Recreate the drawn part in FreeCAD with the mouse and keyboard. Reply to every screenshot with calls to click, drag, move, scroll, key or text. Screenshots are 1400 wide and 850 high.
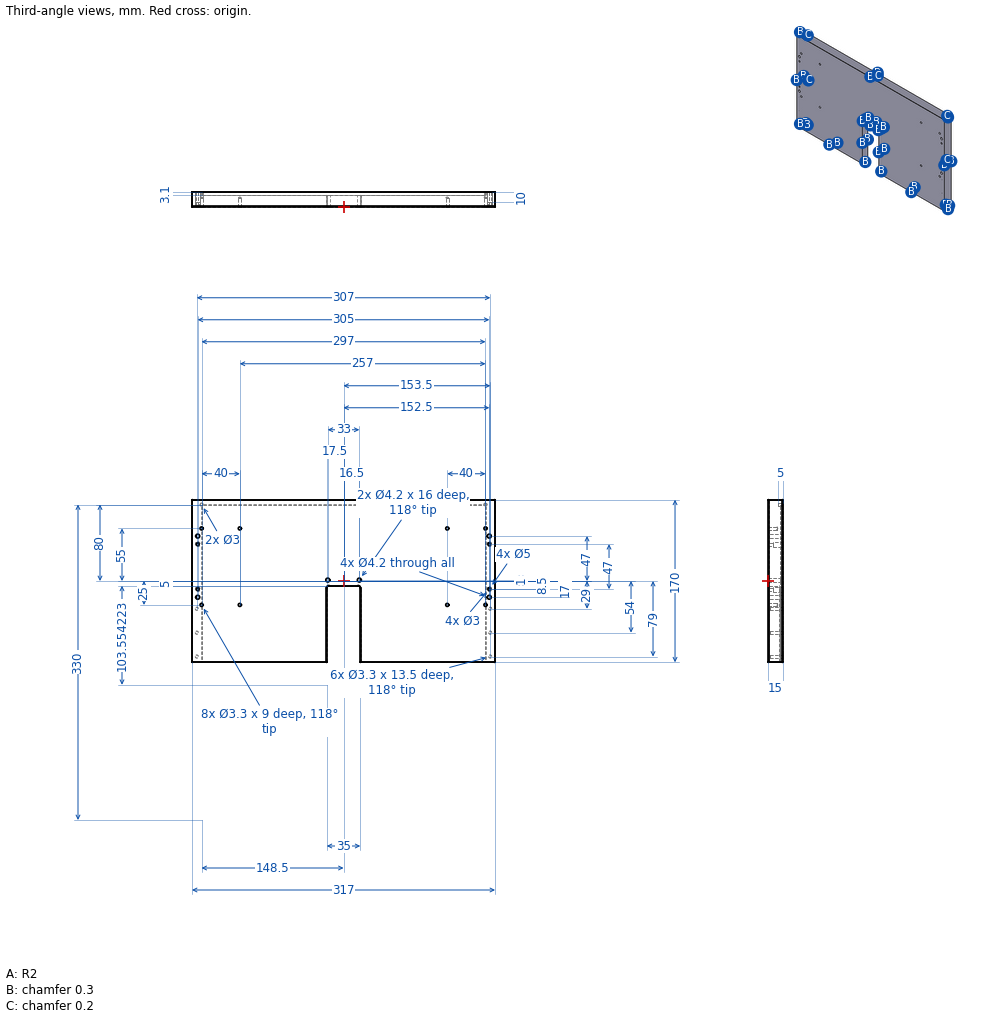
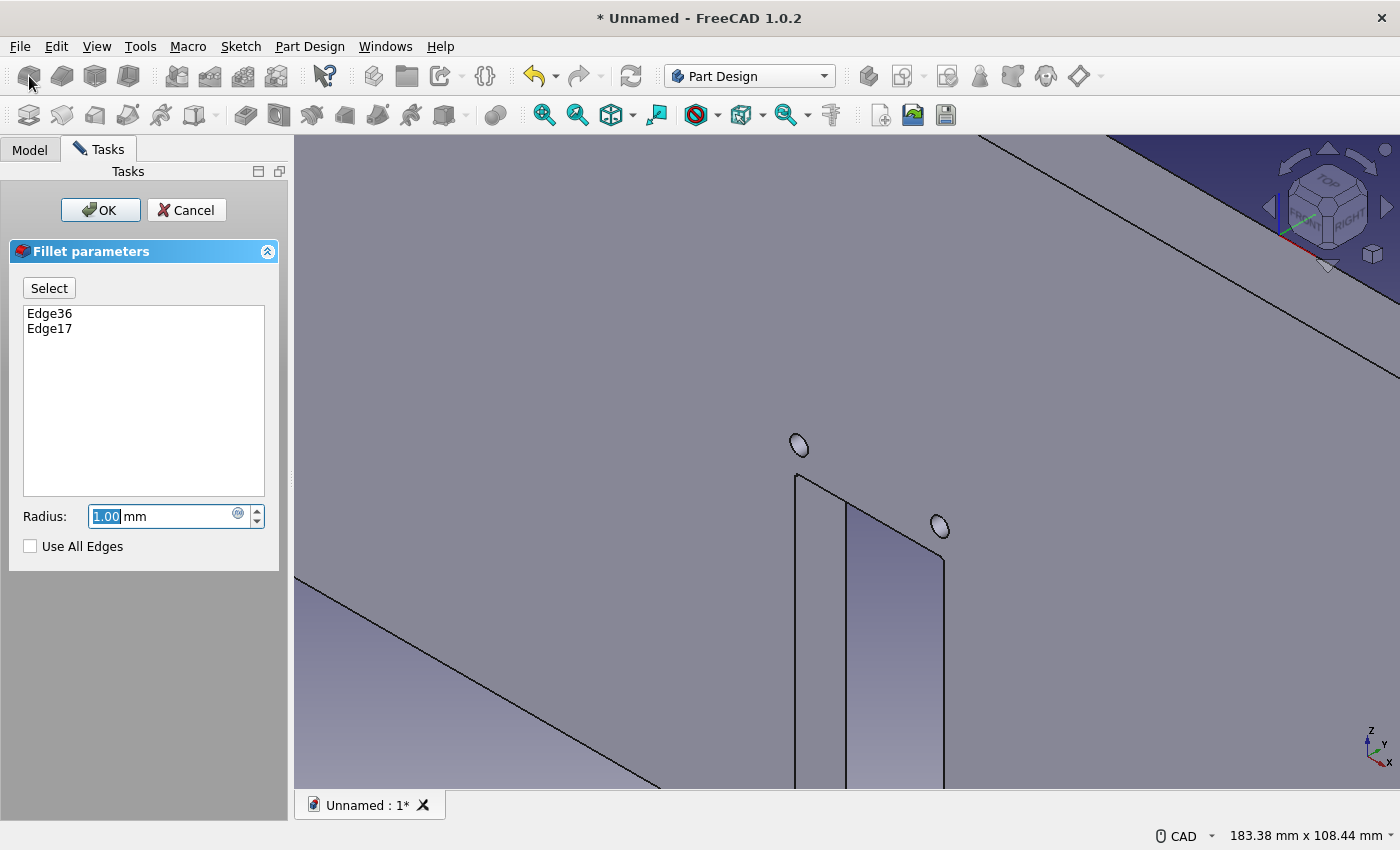
text(2)
key(Tab)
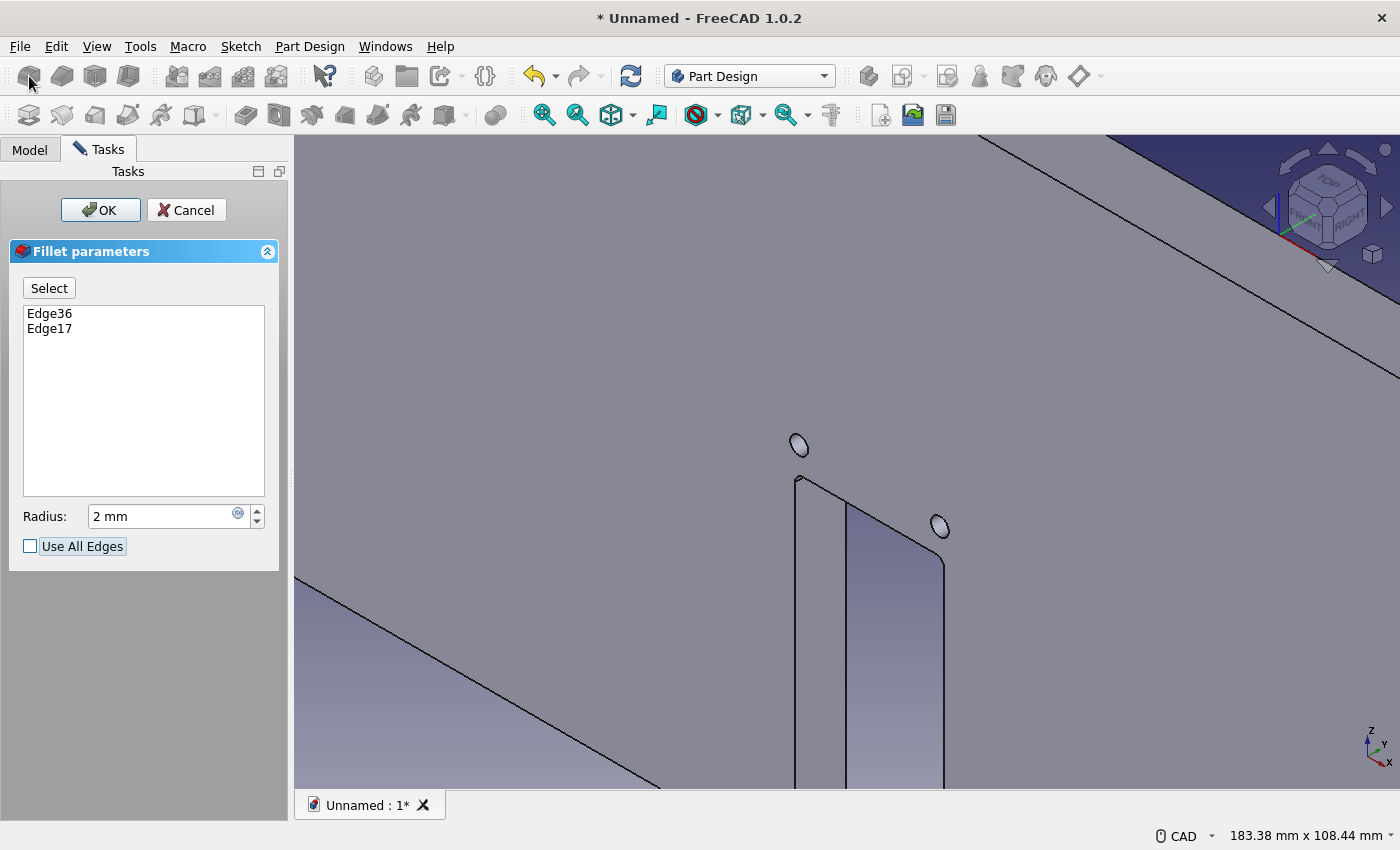
click(101, 210)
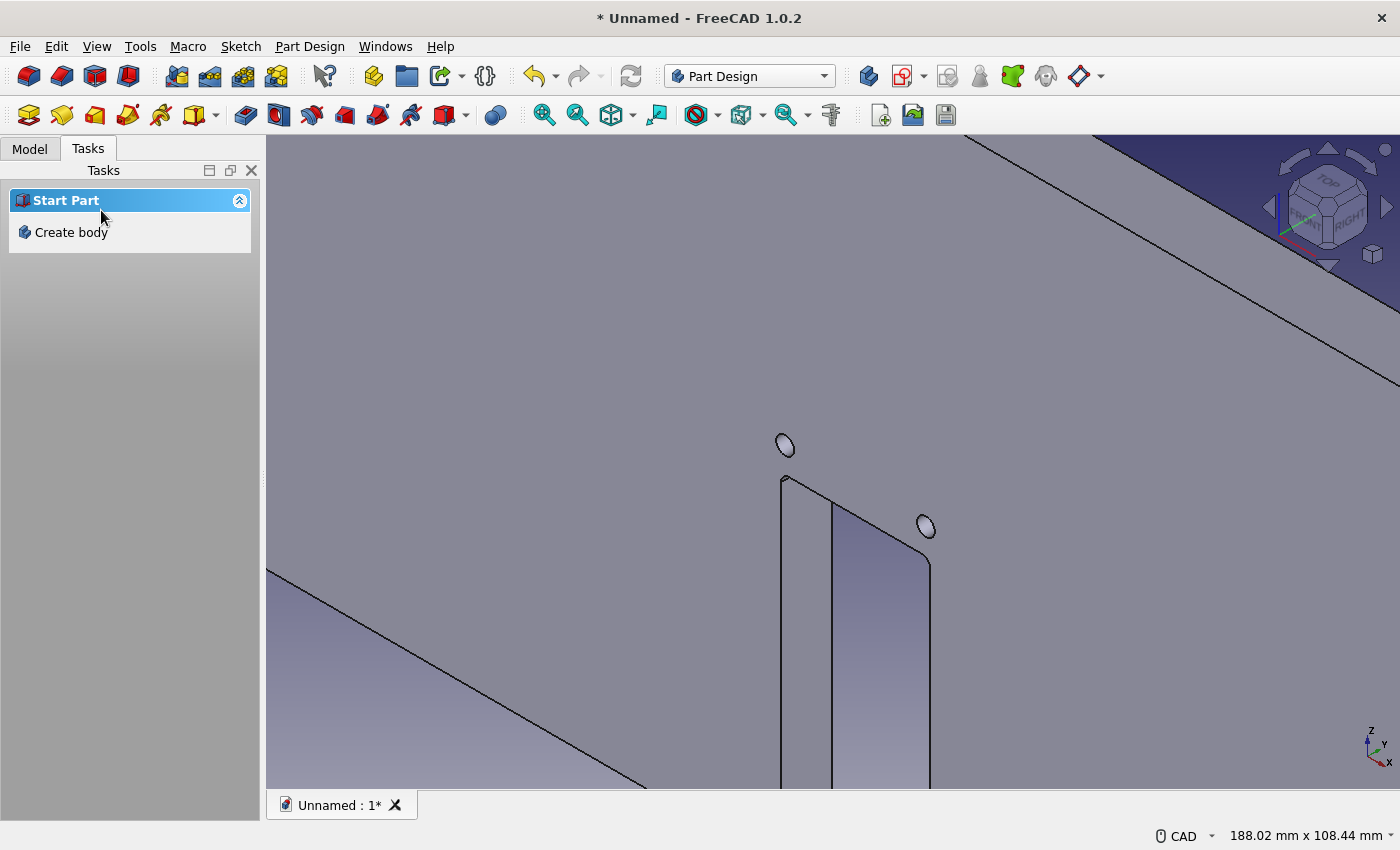
key(v)
key(f)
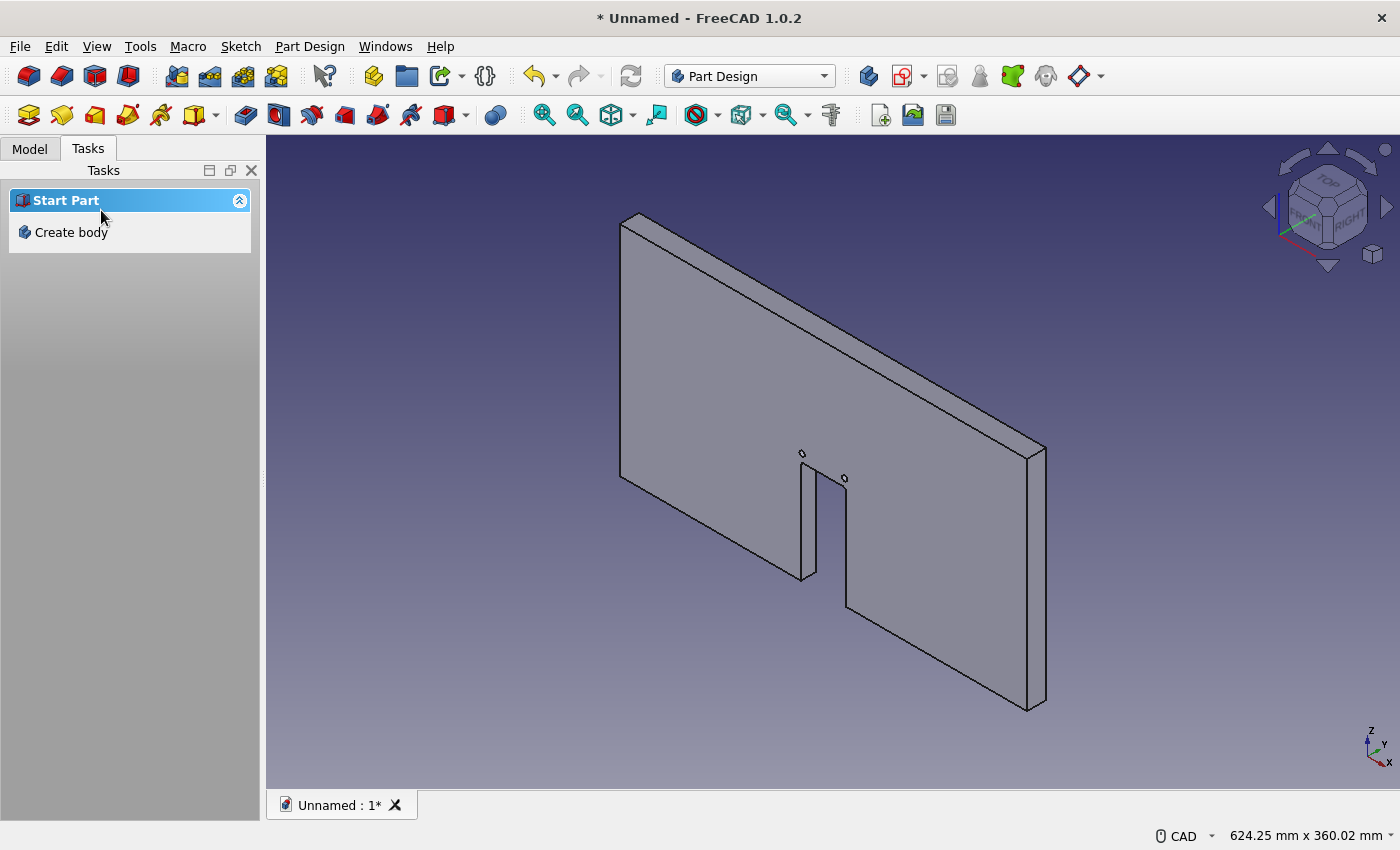
key(4)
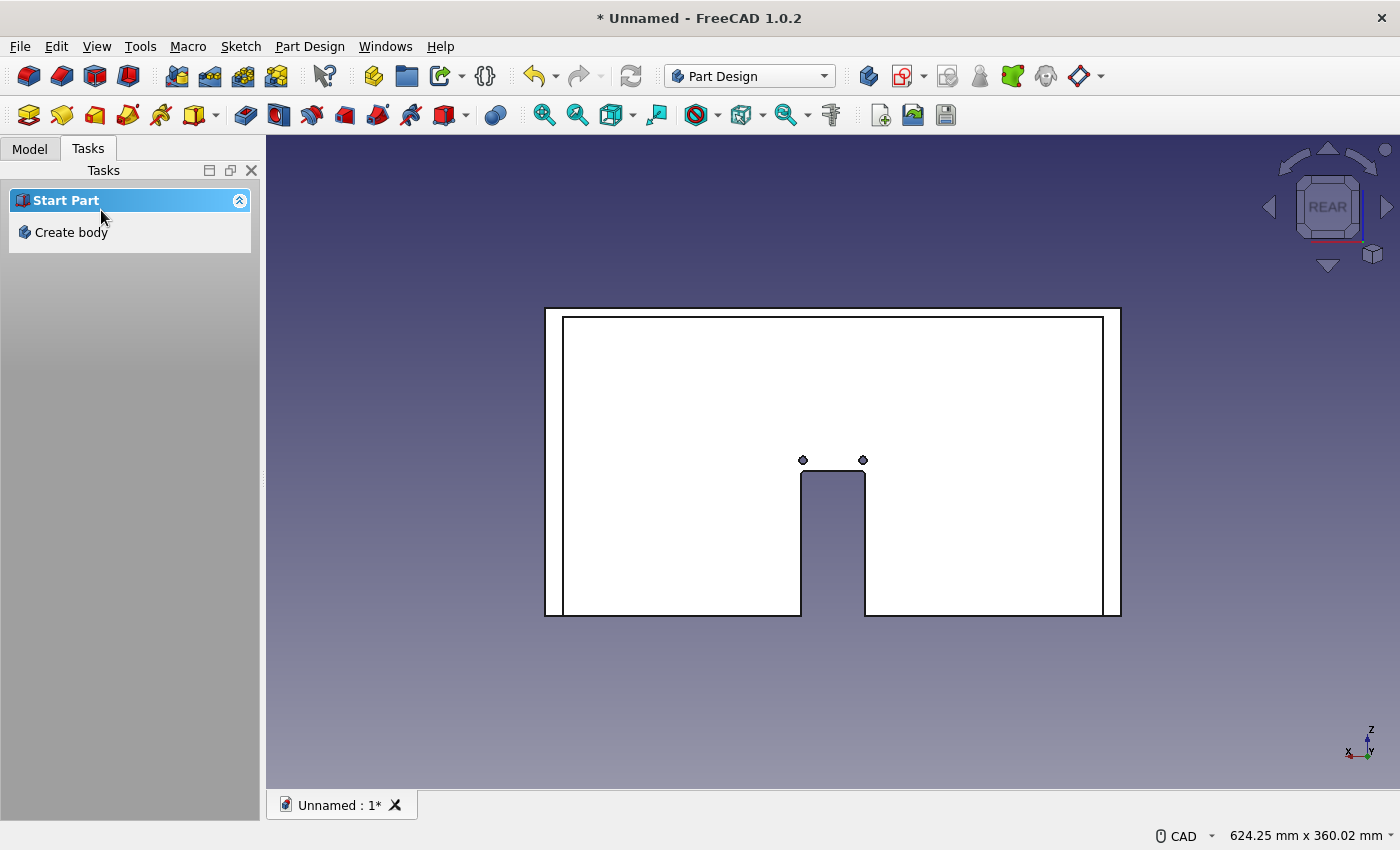
scroll(551, 413, up, 4)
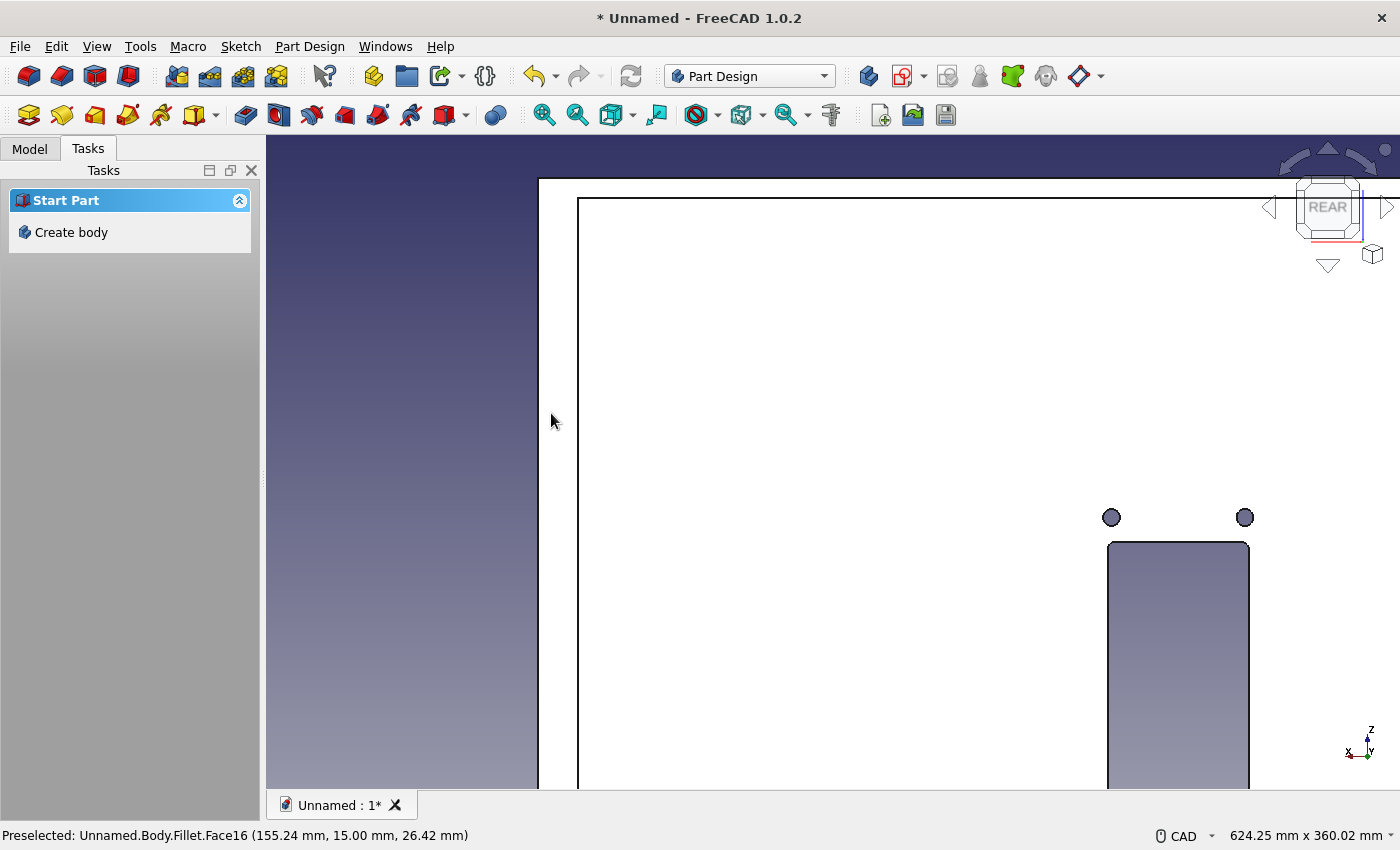
click(551, 413)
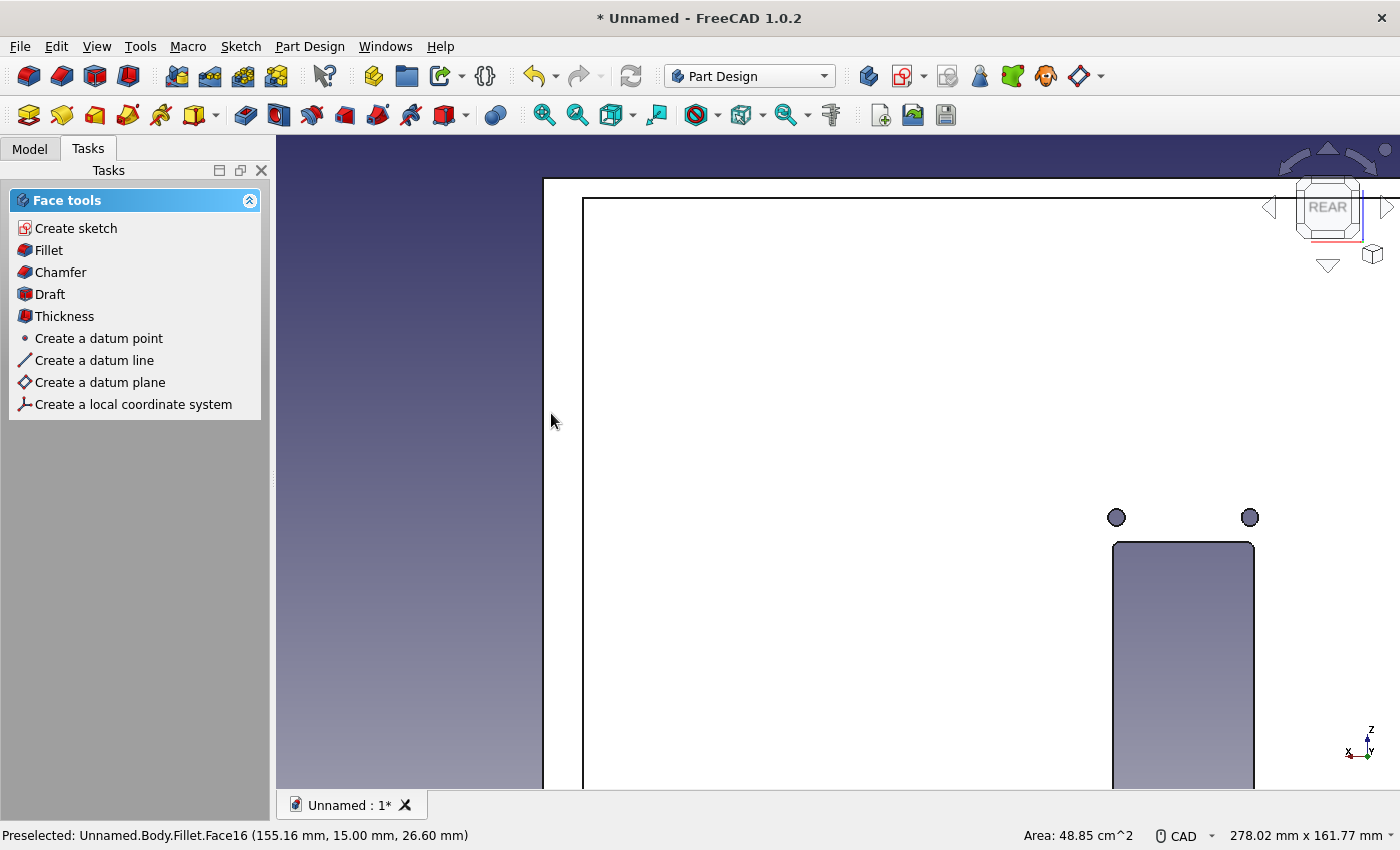
click(902, 76)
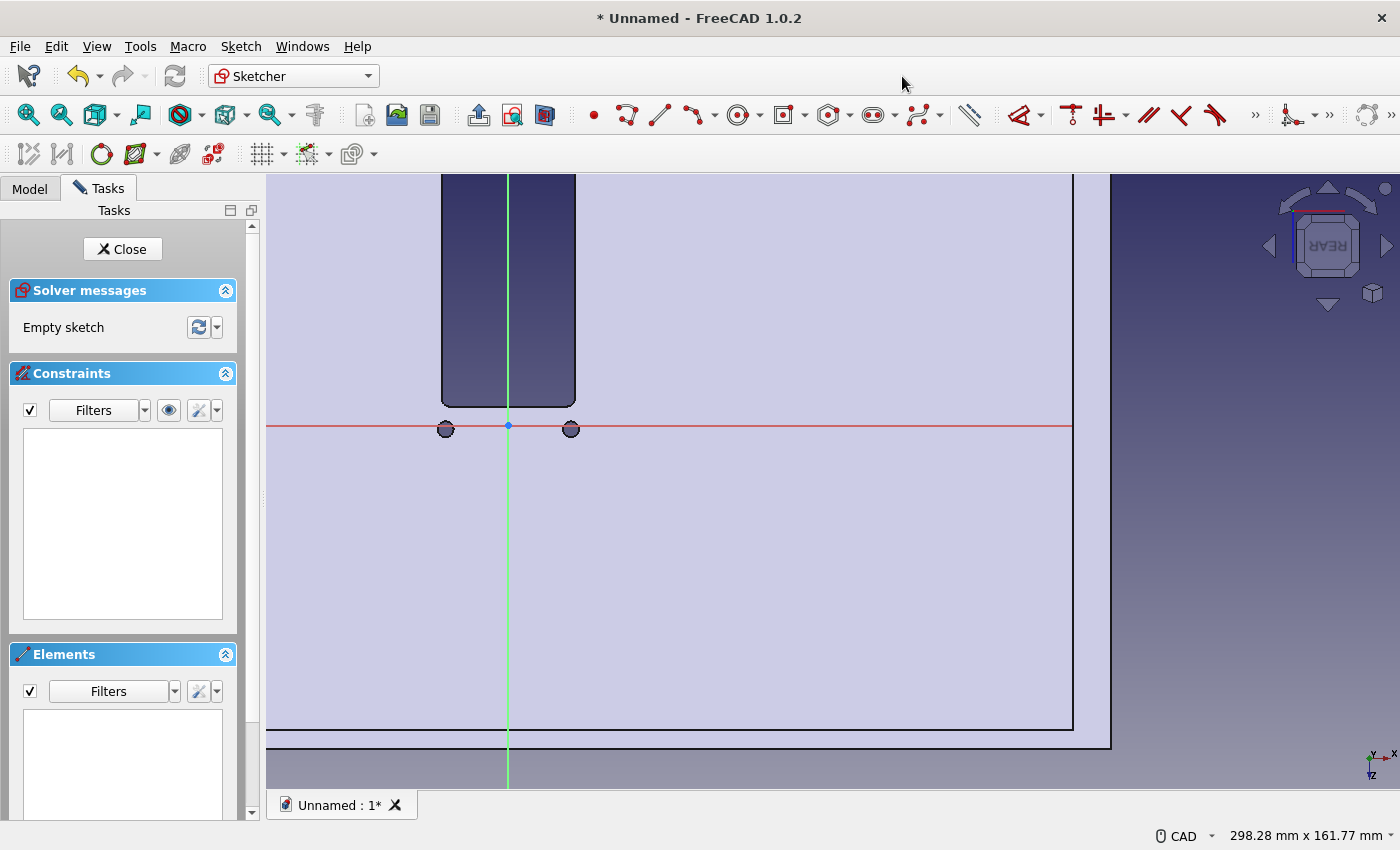
scroll(1076, 361, down, 3)